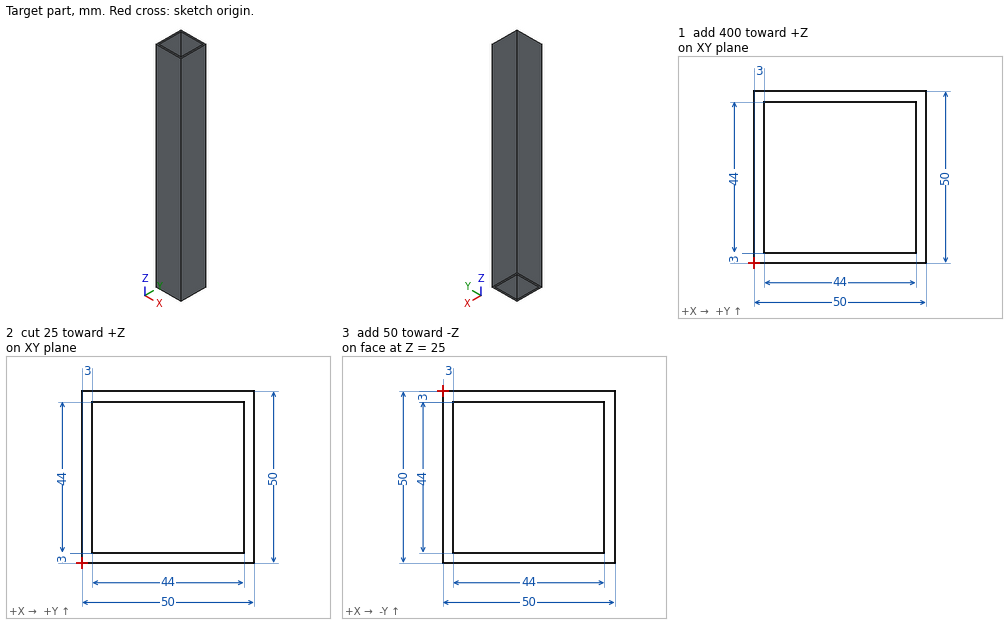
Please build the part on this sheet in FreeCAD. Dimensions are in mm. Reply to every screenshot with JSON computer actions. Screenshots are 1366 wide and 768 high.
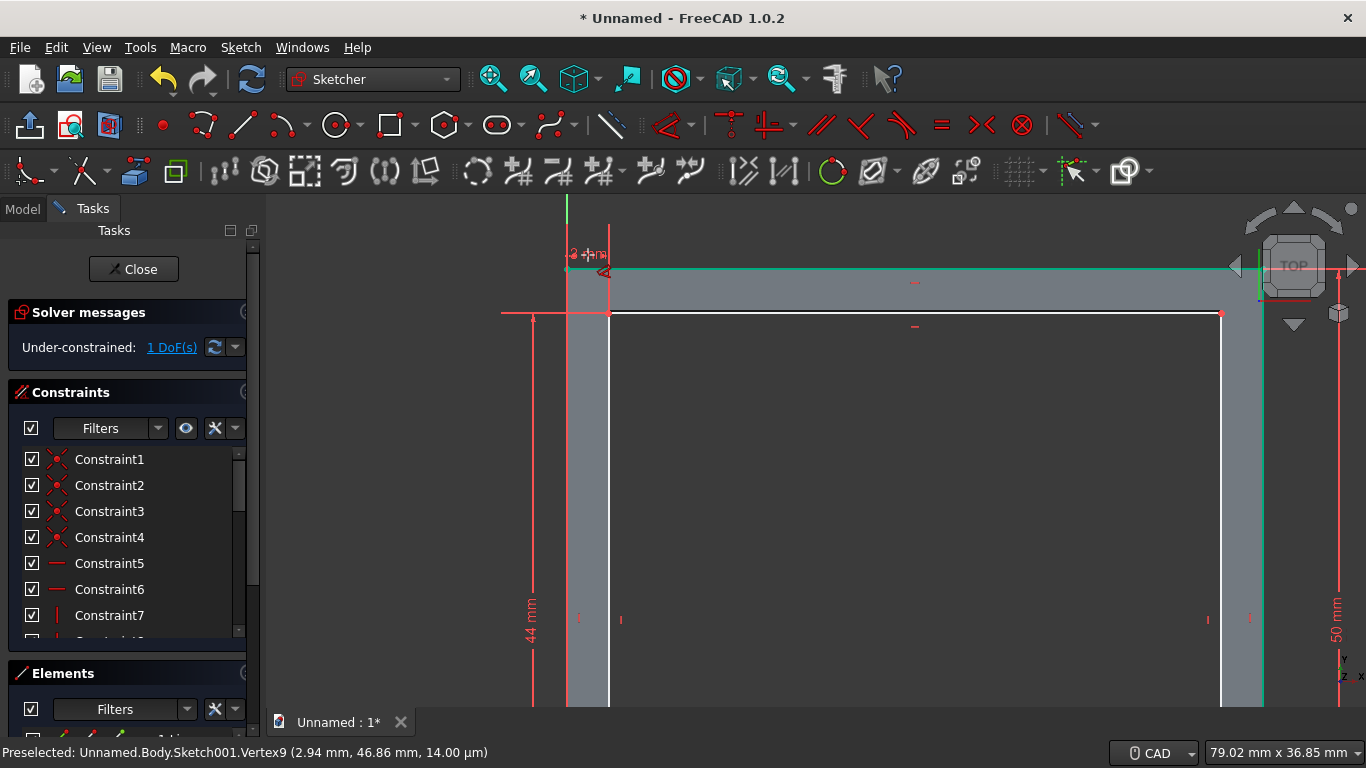
{"action": "scroll", "coordinate": [611, 314], "scroll_direction": "down", "scroll_amount": 4}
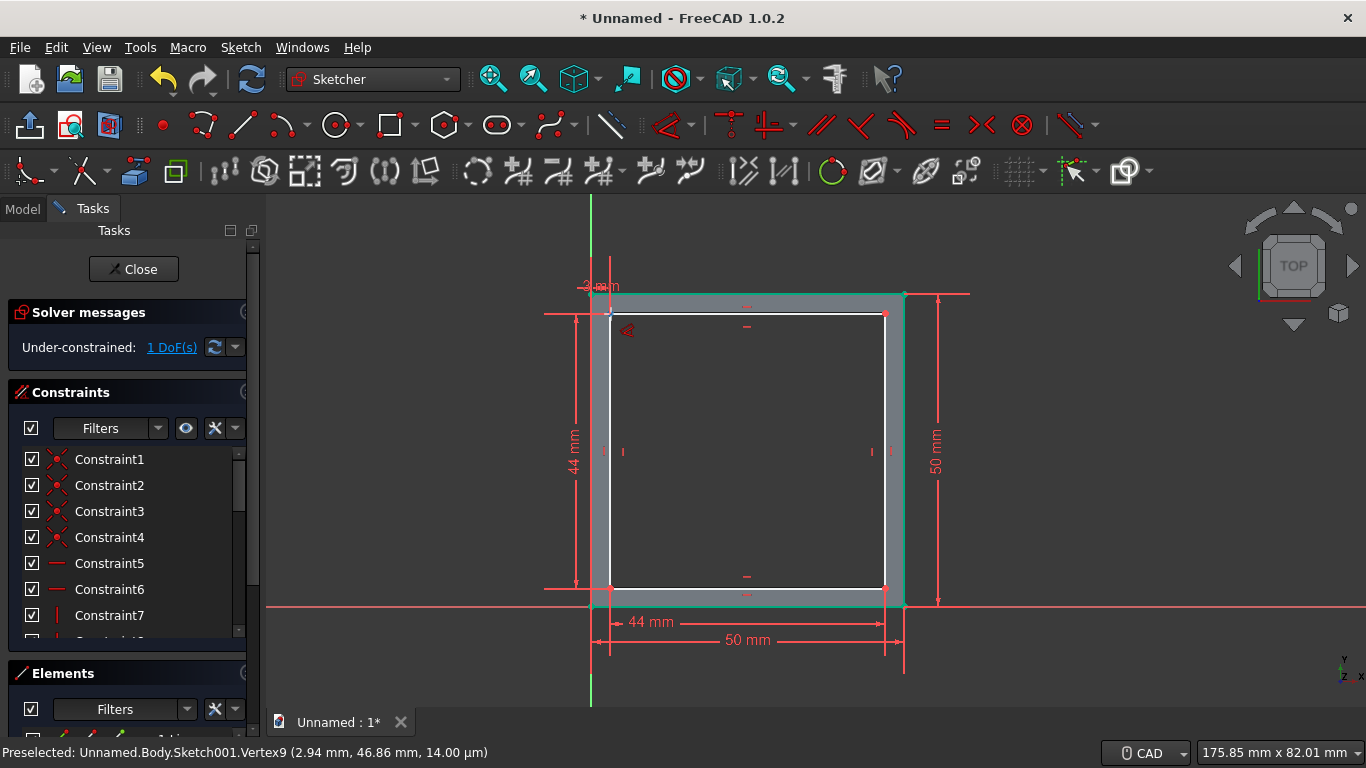
{"action": "scroll", "coordinate": [610, 589], "scroll_direction": "up", "scroll_amount": 4}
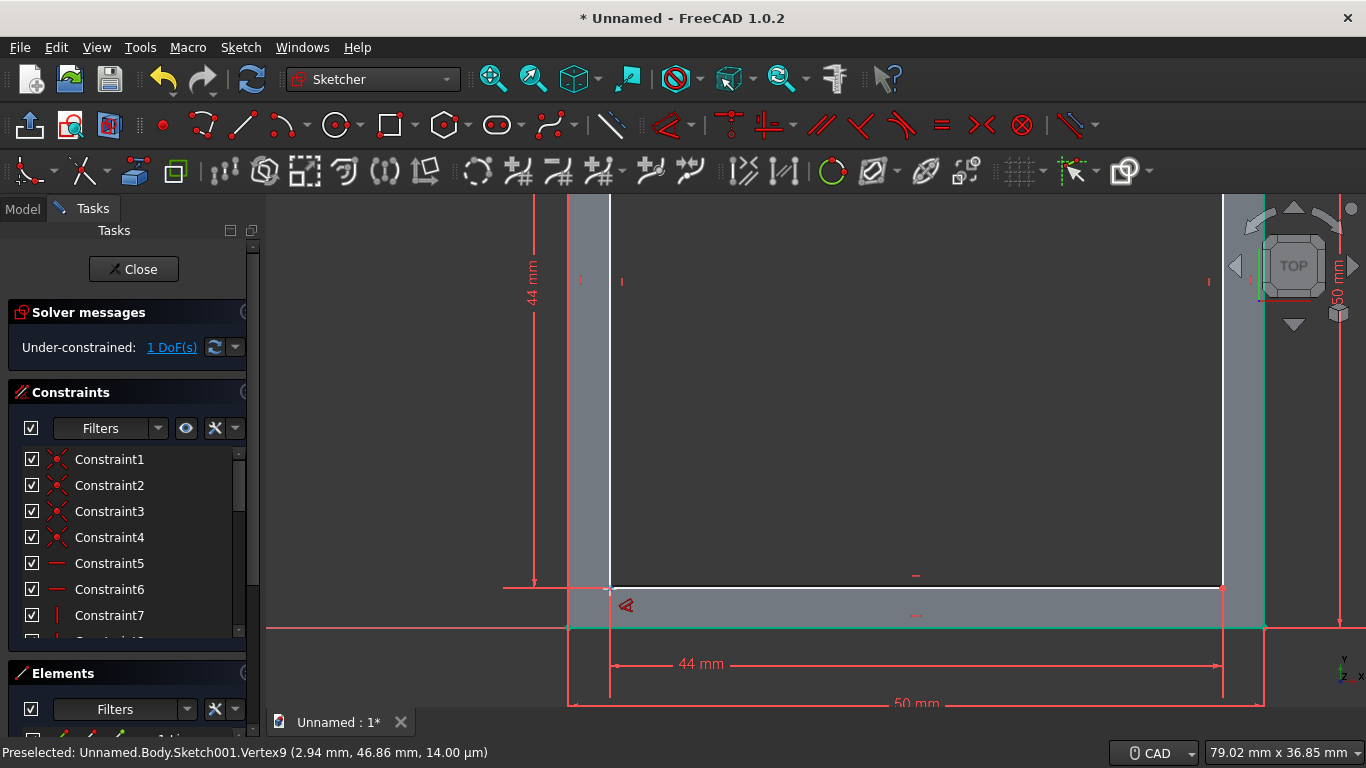
{"action": "left_click", "coordinate": [610, 588]}
{"action": "left_click", "coordinate": [534, 608]}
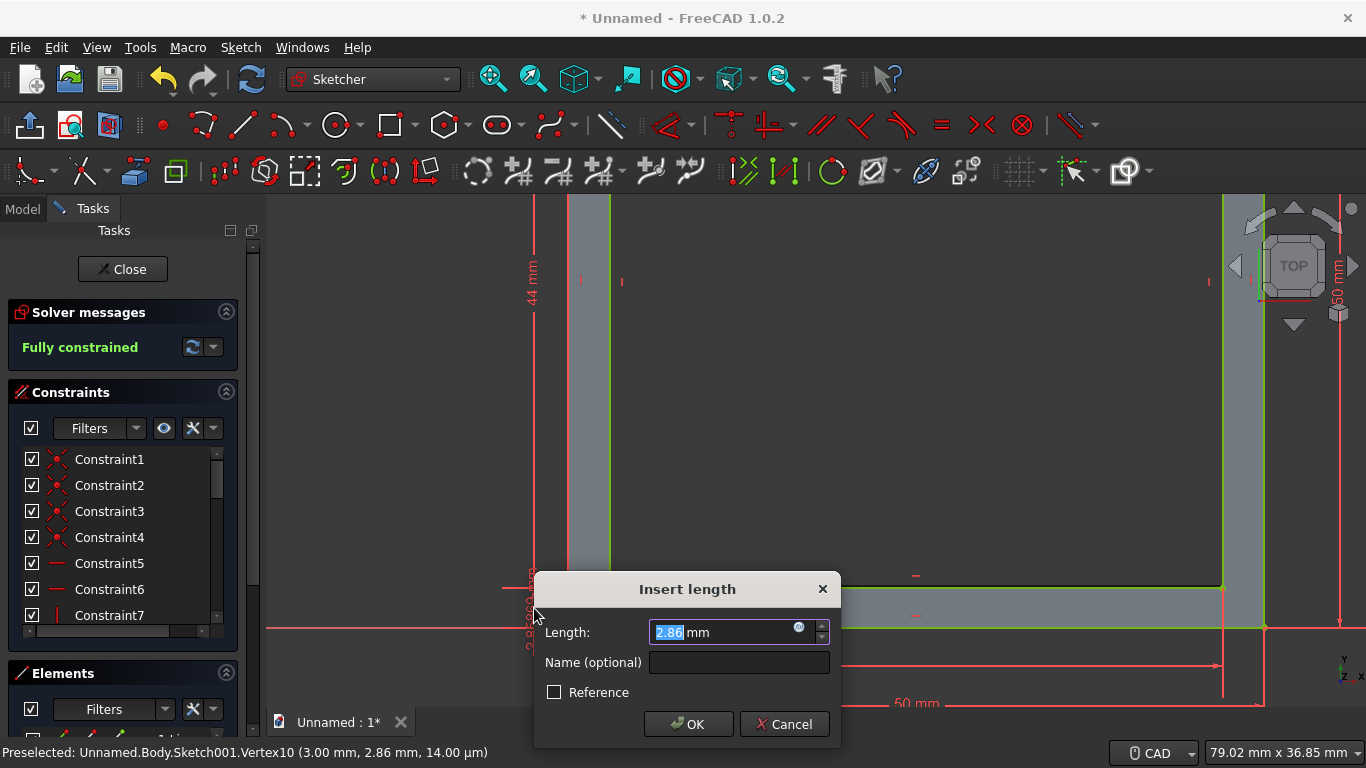
{"action": "type", "text": "3"}
{"action": "key", "text": "Return"}
{"action": "key", "text": "Escape"}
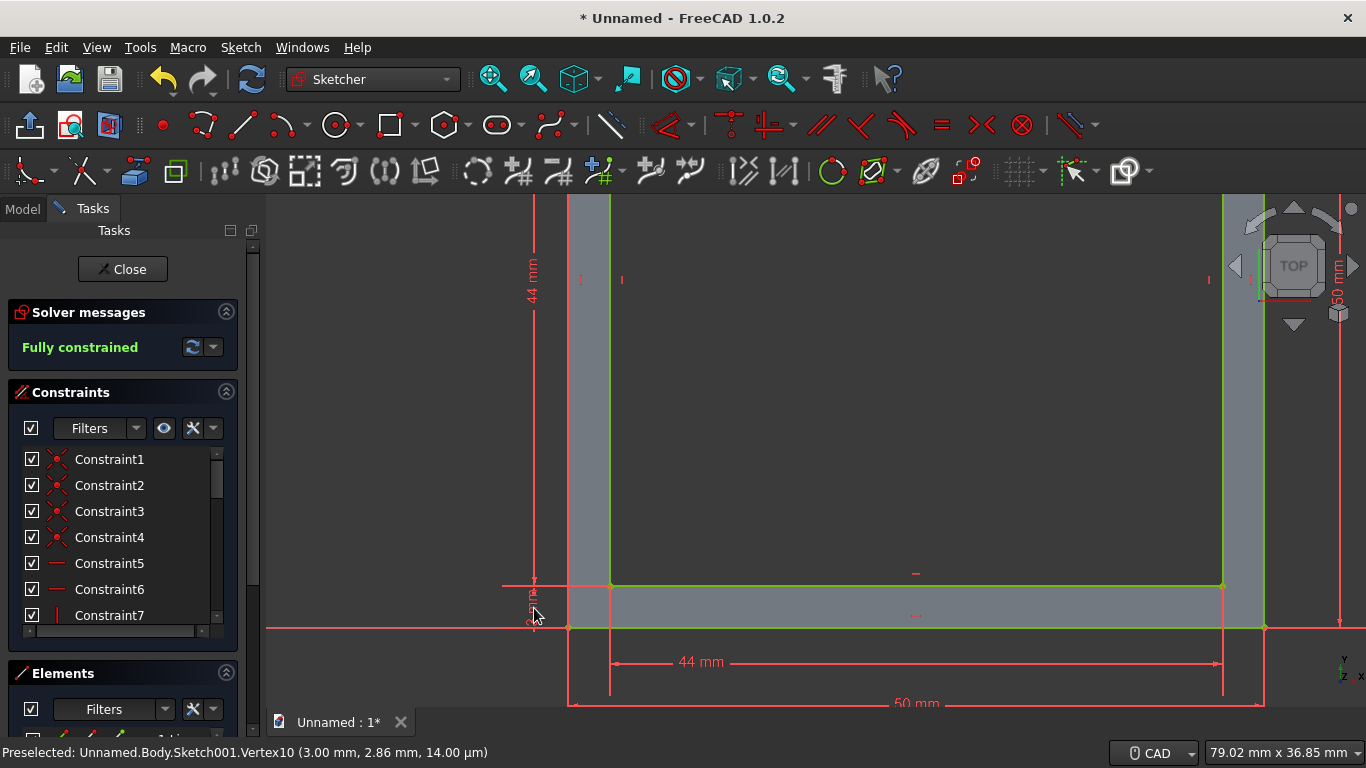
{"action": "left_click", "coordinate": [123, 269]}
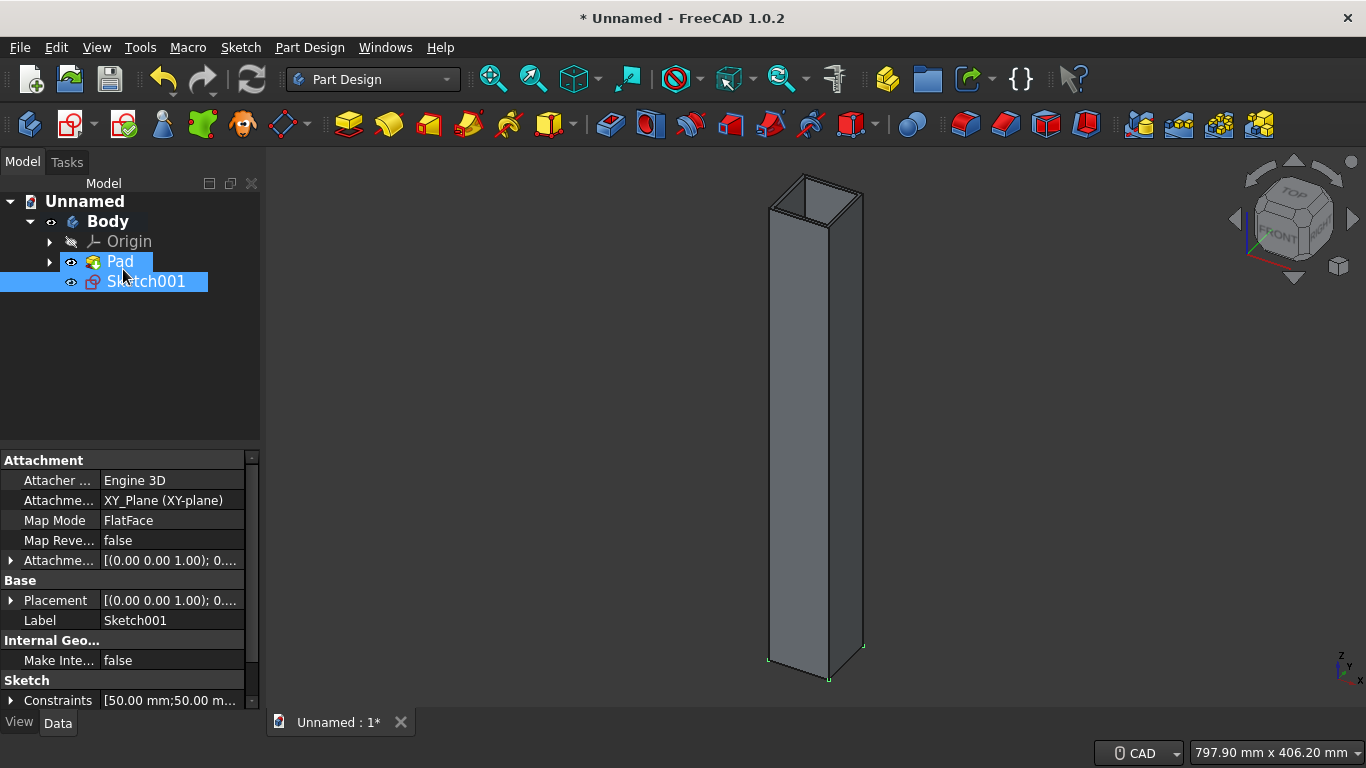
{"action": "left_click", "coordinate": [612, 124]}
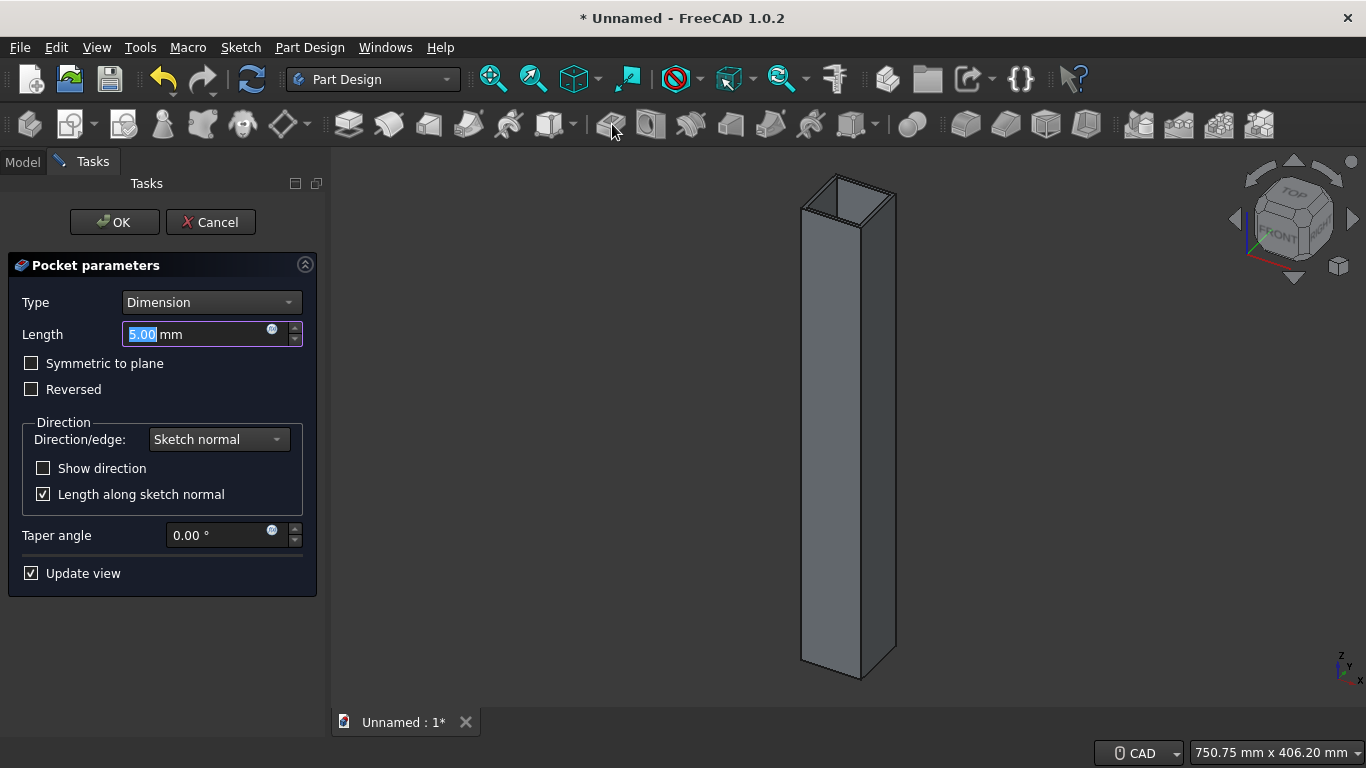
{"action": "type", "text": "25"}
{"action": "key", "text": "Tab"}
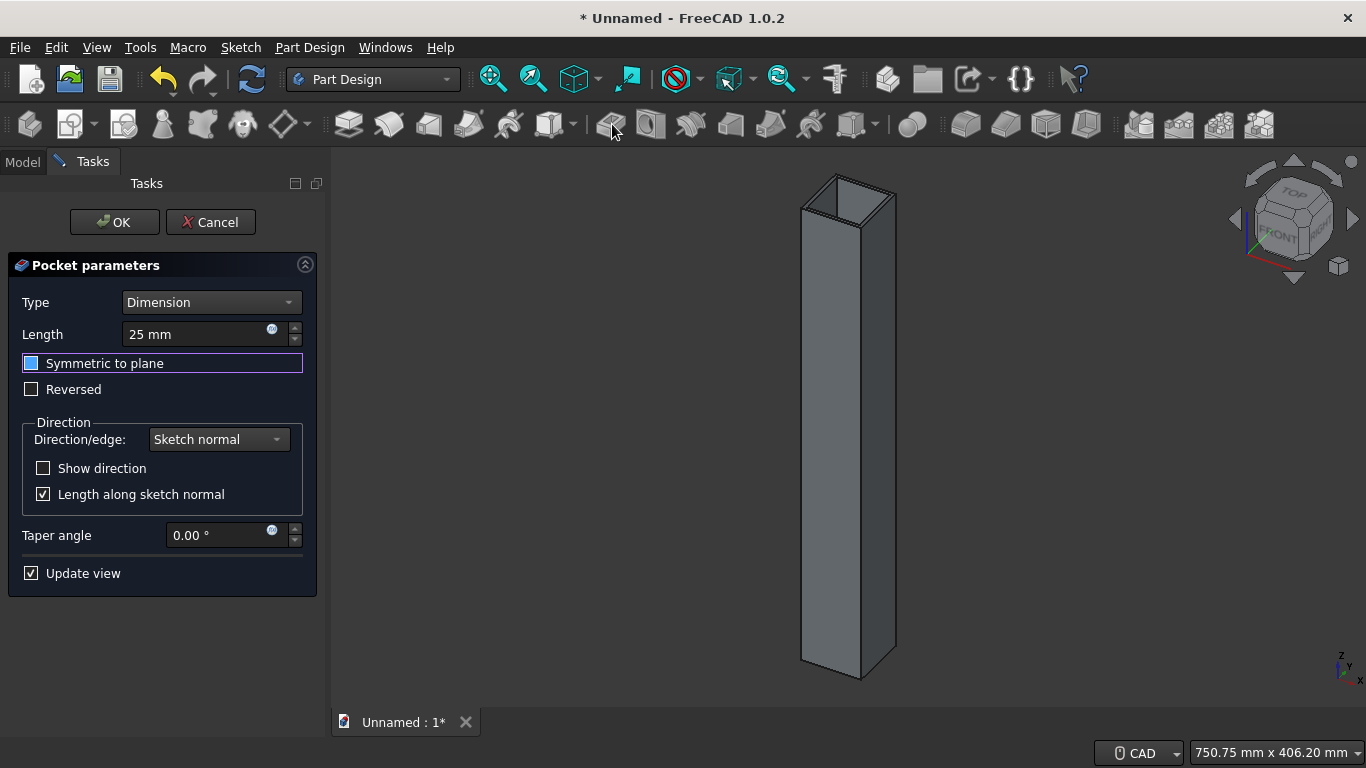
{"action": "left_click", "coordinate": [30, 389]}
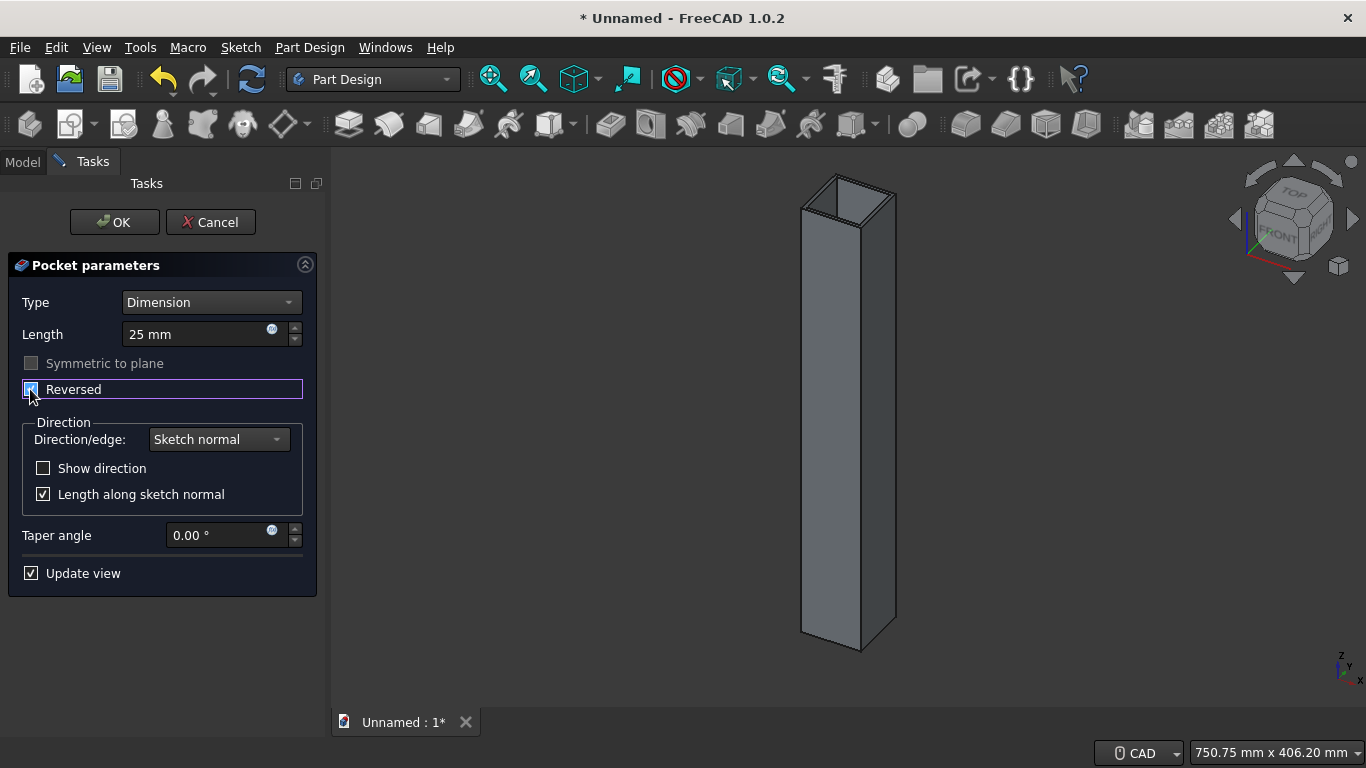
{"action": "left_click", "coordinate": [115, 222]}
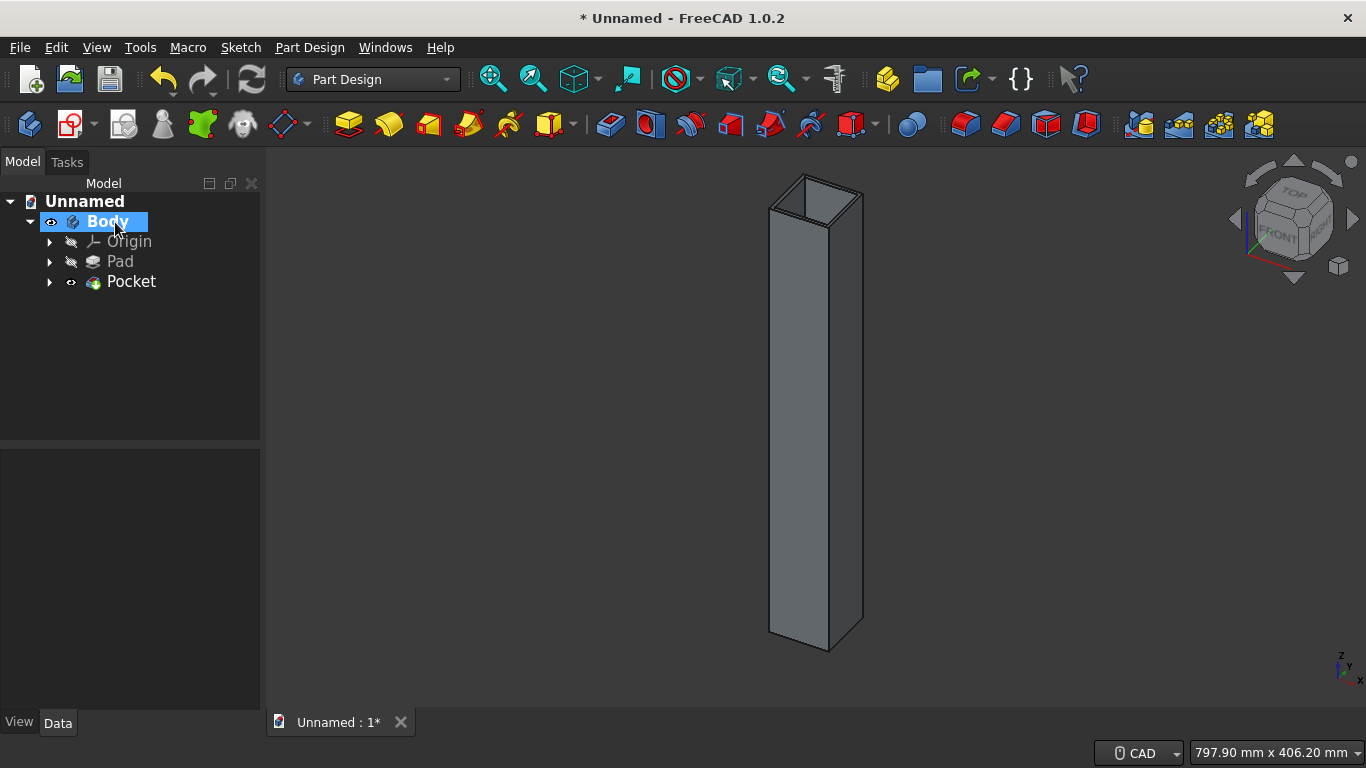
{"action": "key", "text": "5"}